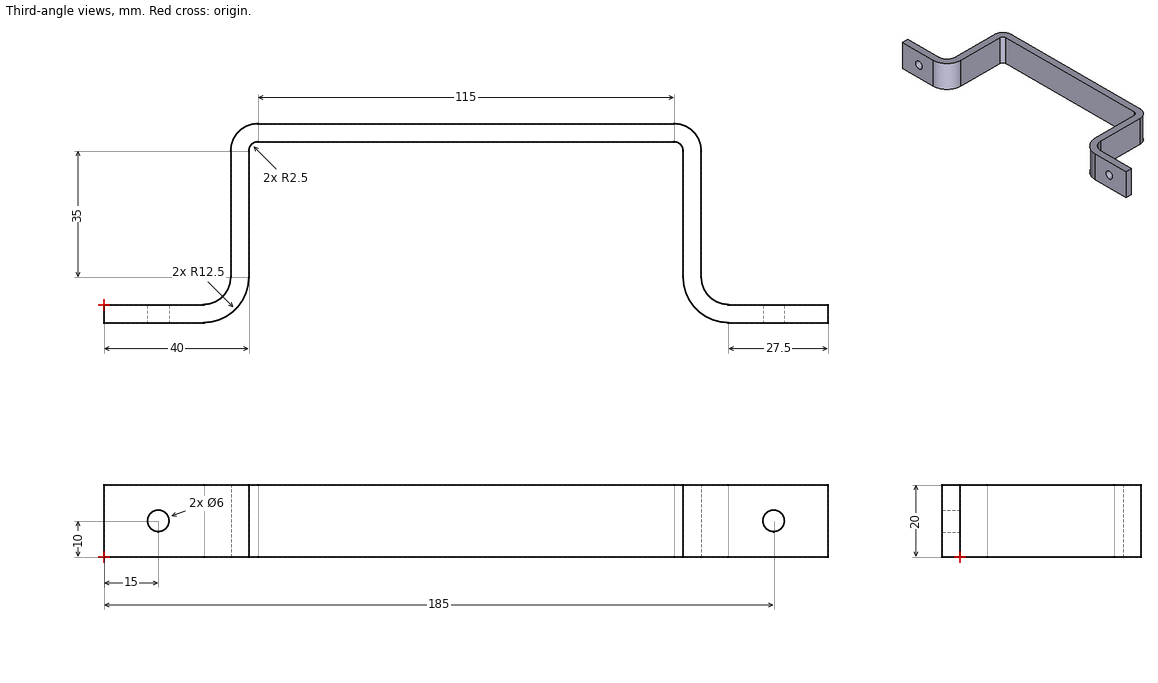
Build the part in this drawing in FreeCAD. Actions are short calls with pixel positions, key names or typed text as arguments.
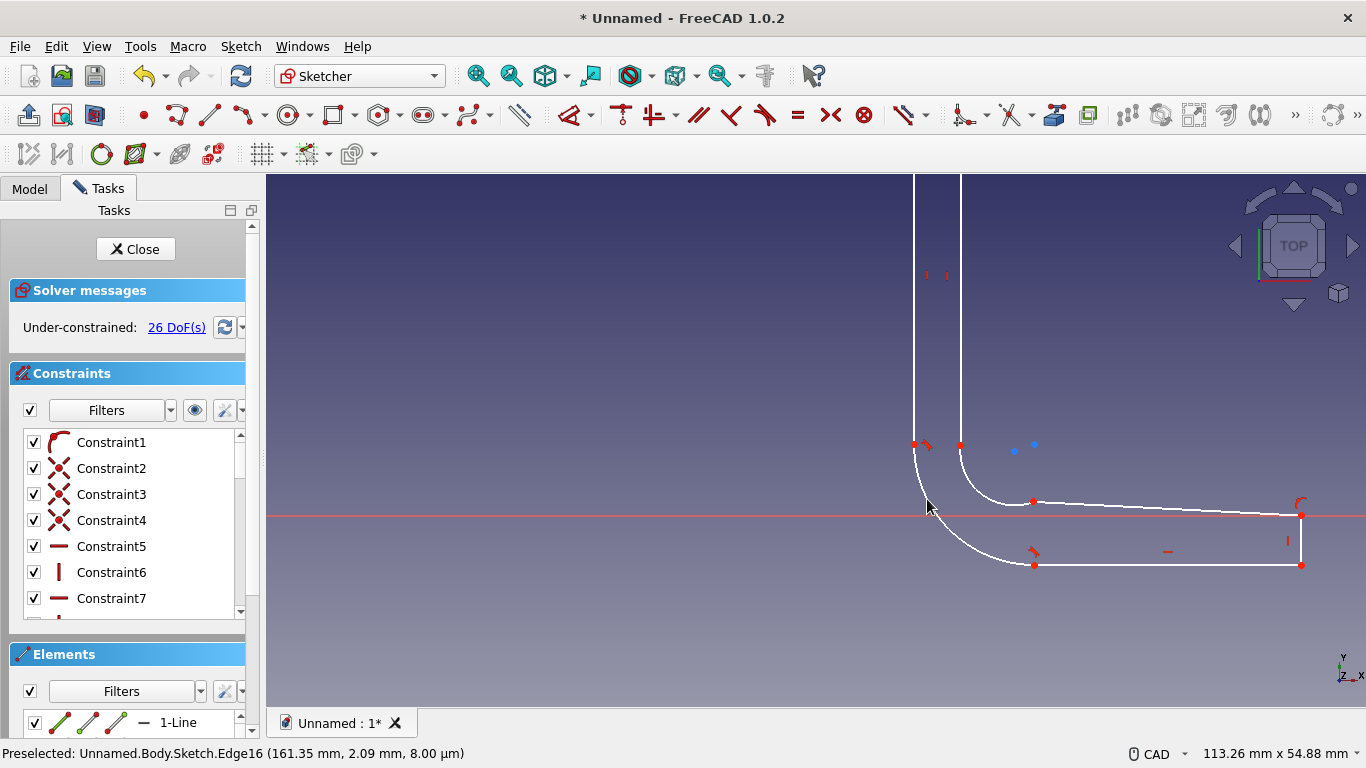
scroll(1114, 506, up, 2)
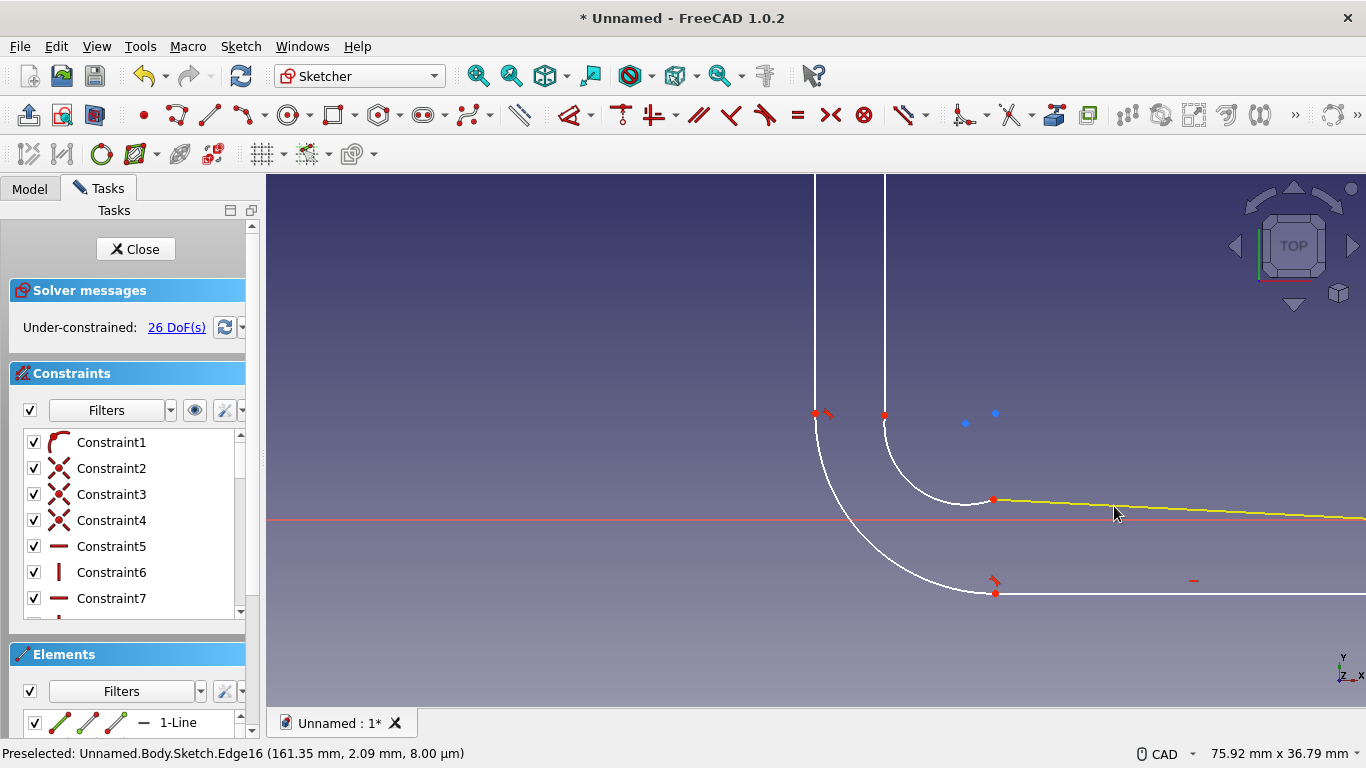
click(1113, 506)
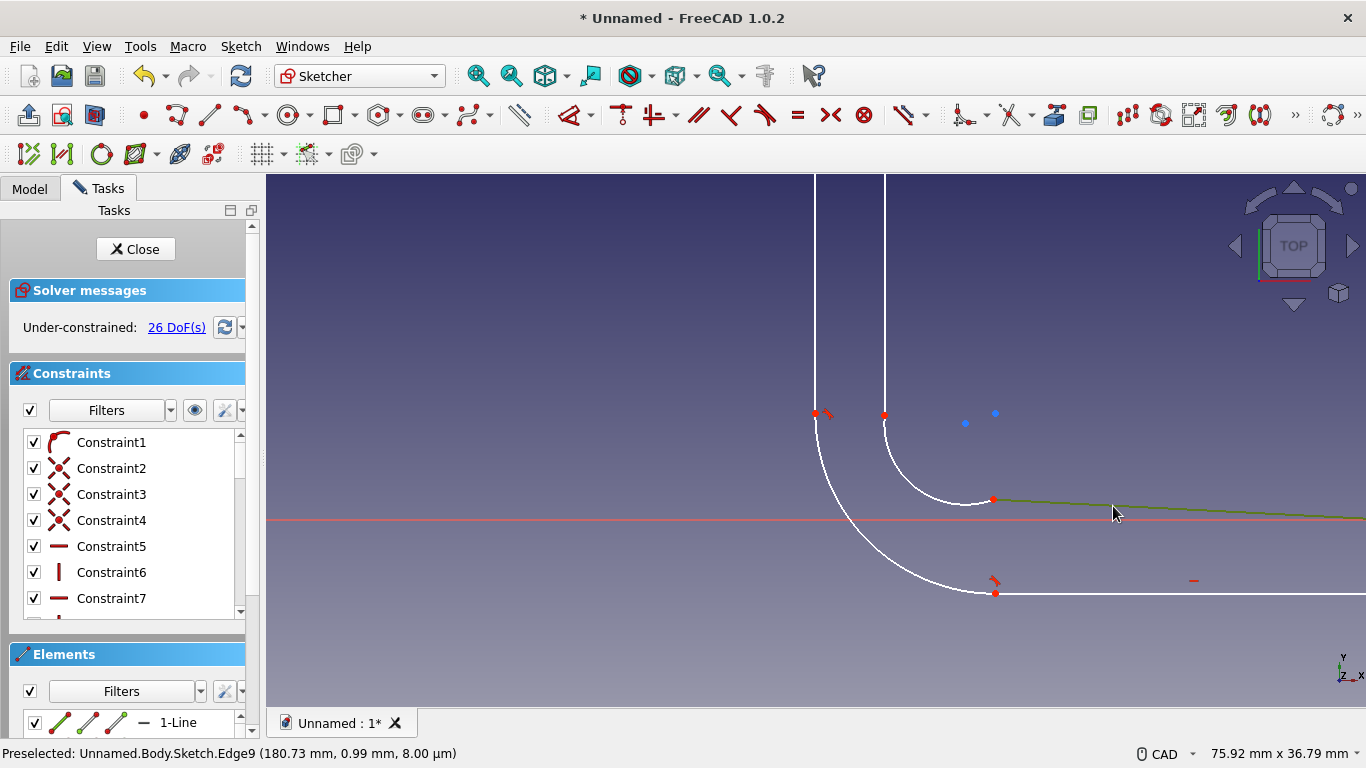
scroll(951, 503, down, 8)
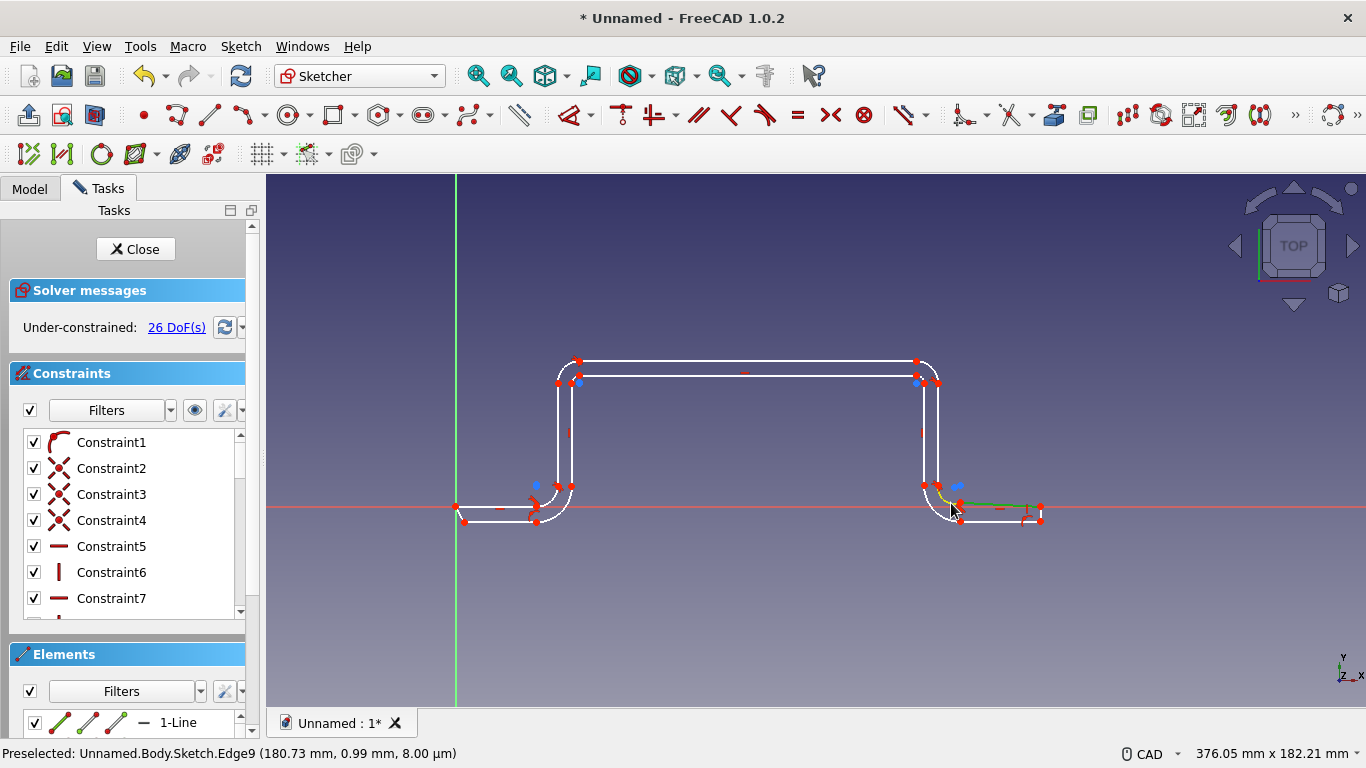
scroll(940, 495, up, 2)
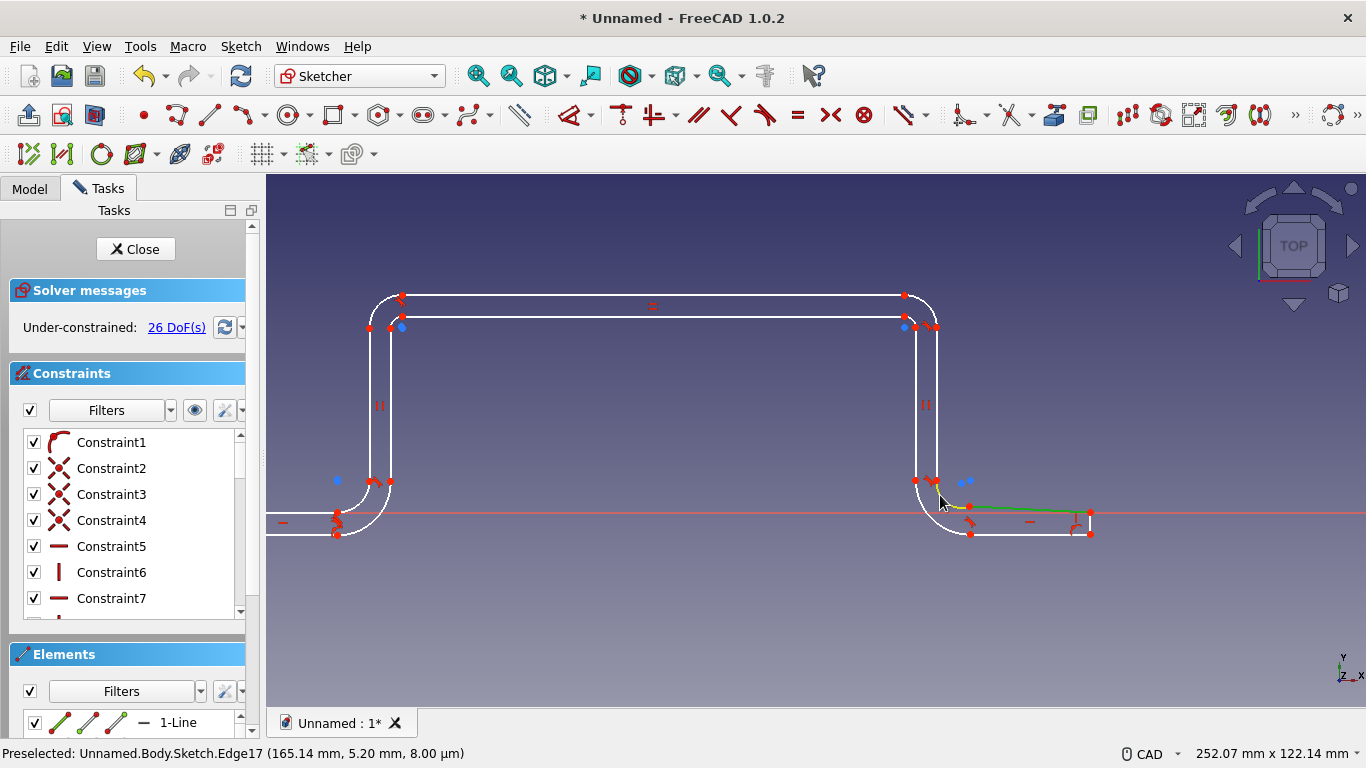
click(940, 495)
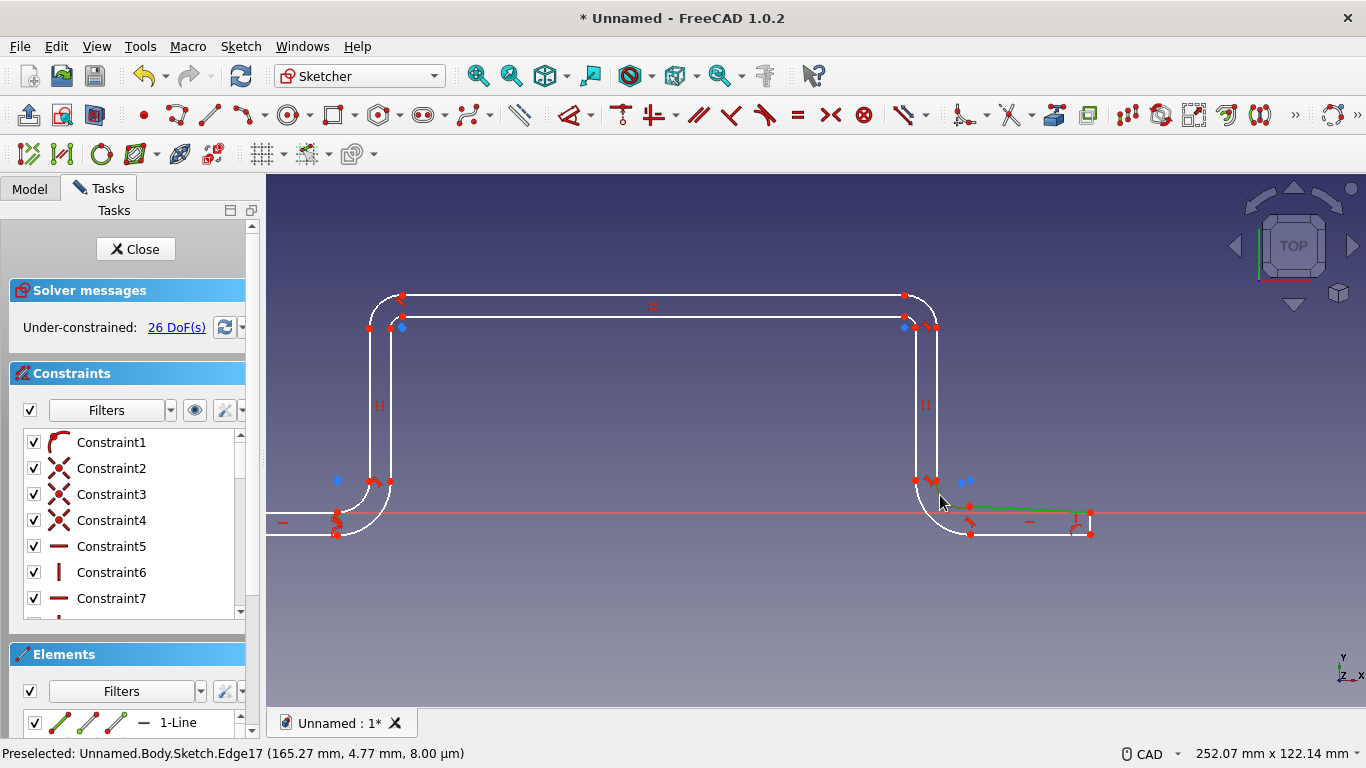
click(765, 116)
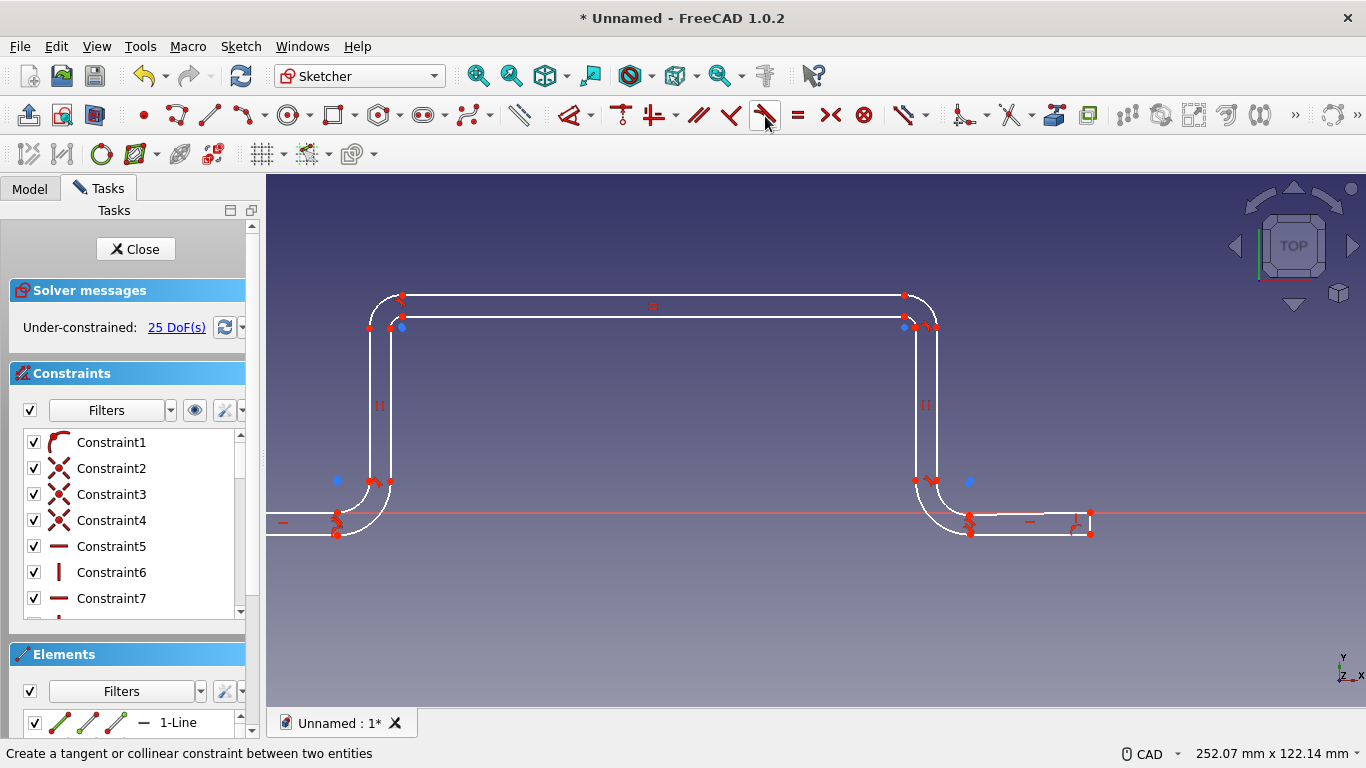
click(937, 435)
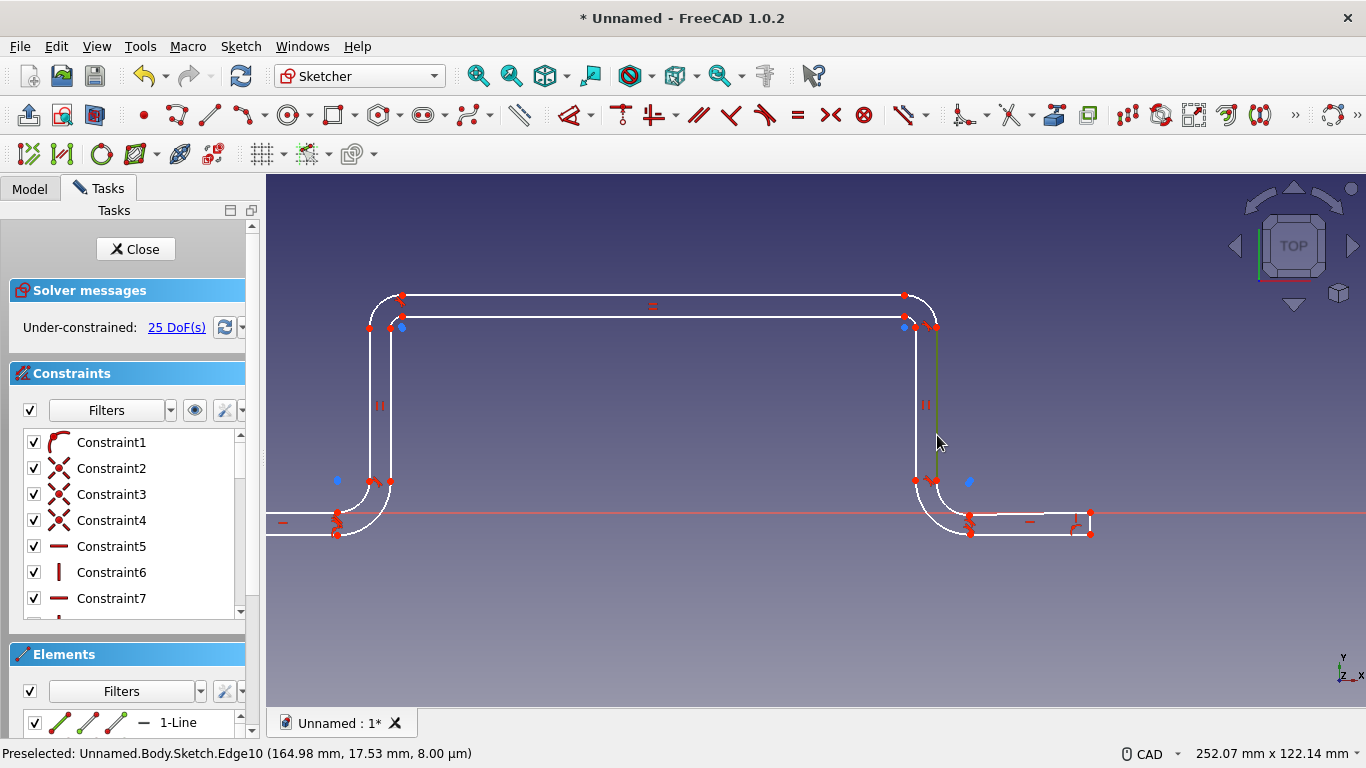
click(940, 496)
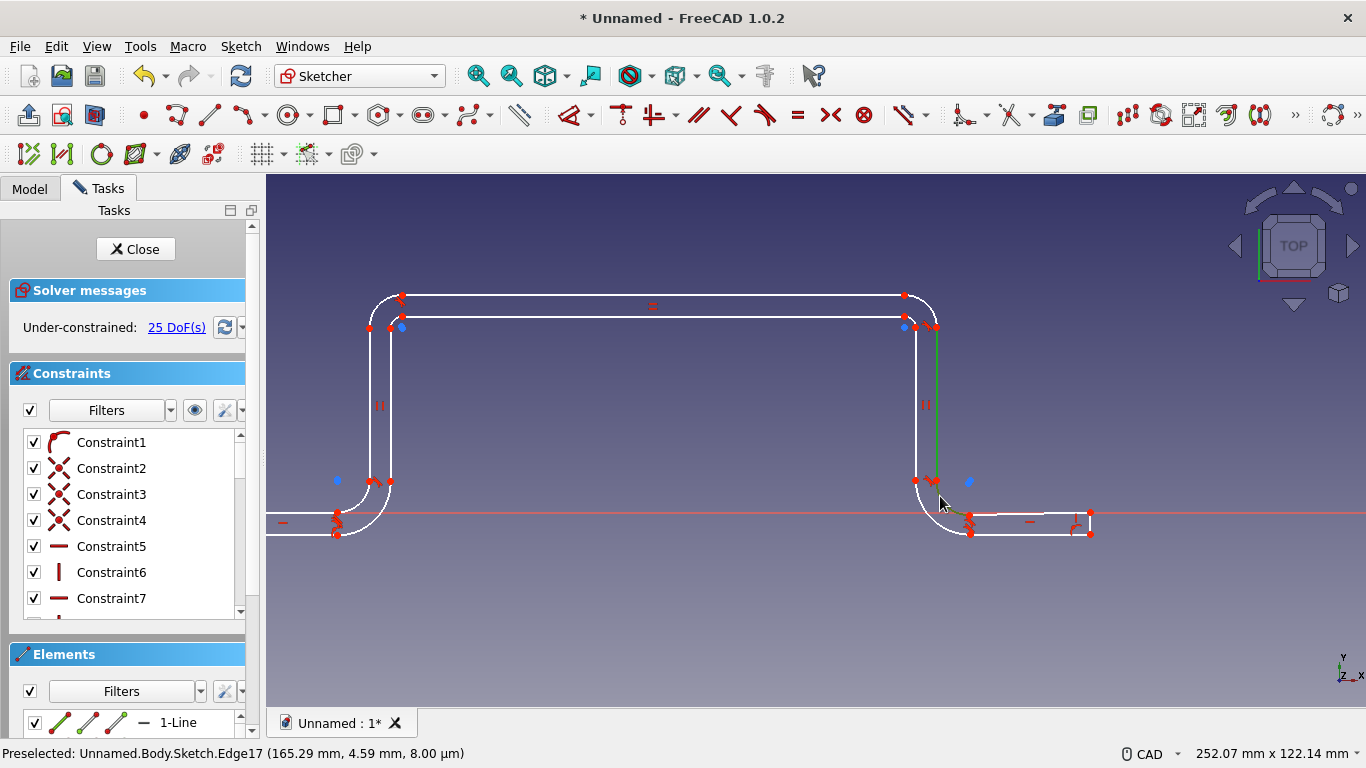
click(765, 116)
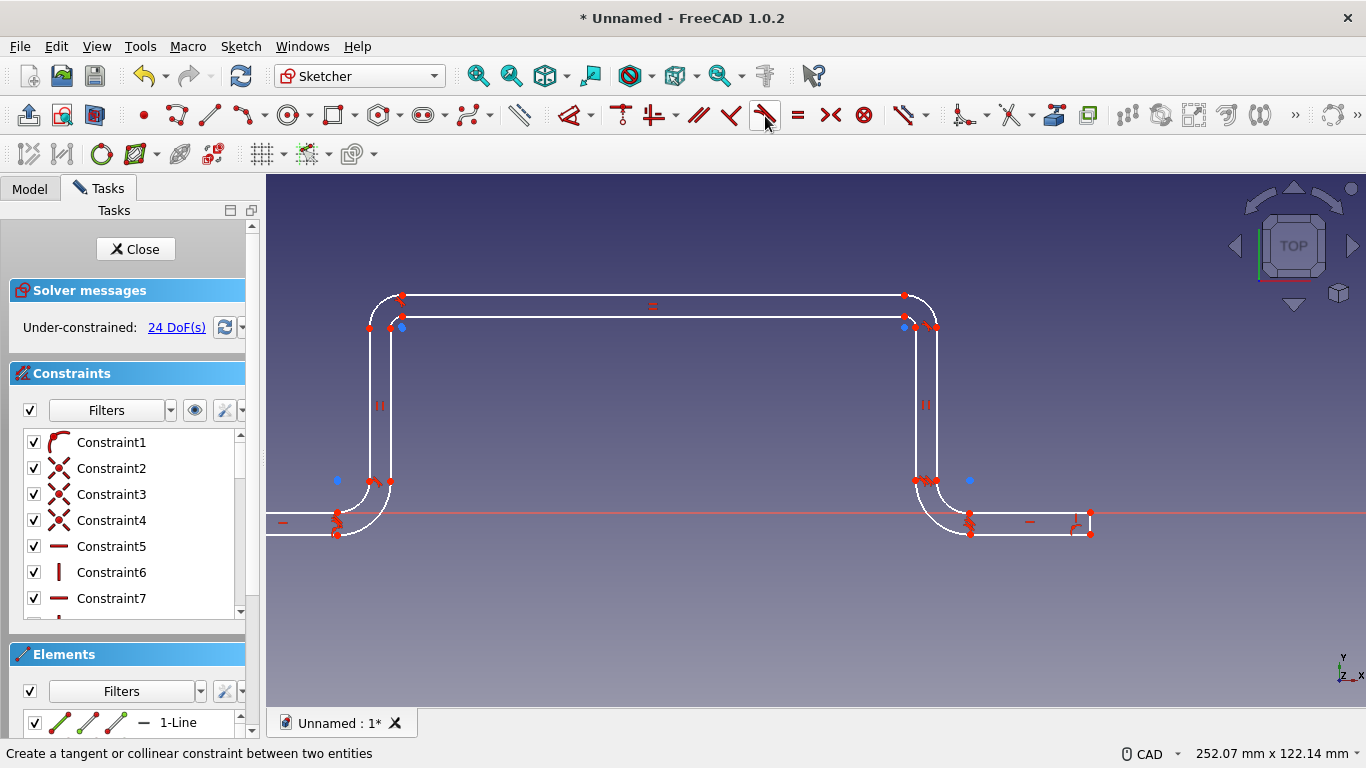
click(937, 435)